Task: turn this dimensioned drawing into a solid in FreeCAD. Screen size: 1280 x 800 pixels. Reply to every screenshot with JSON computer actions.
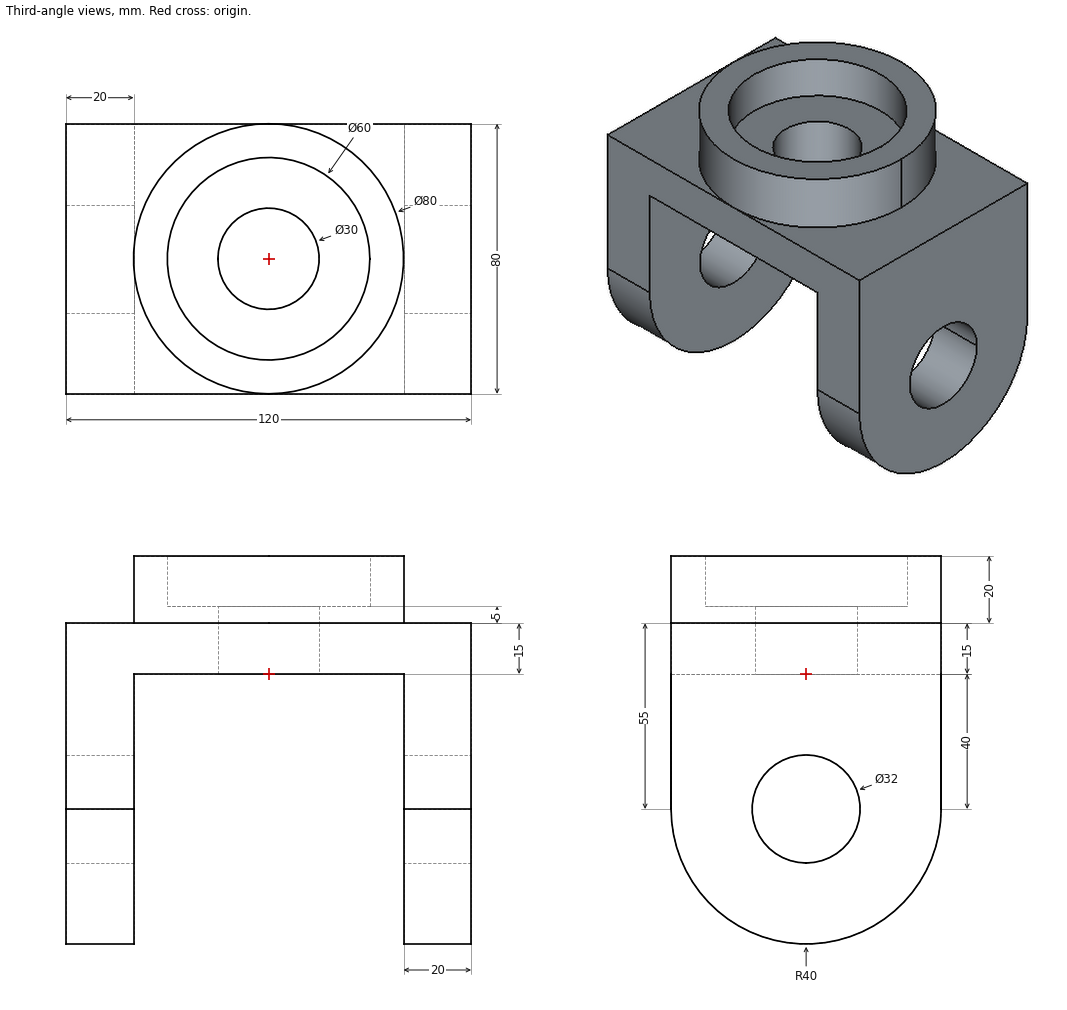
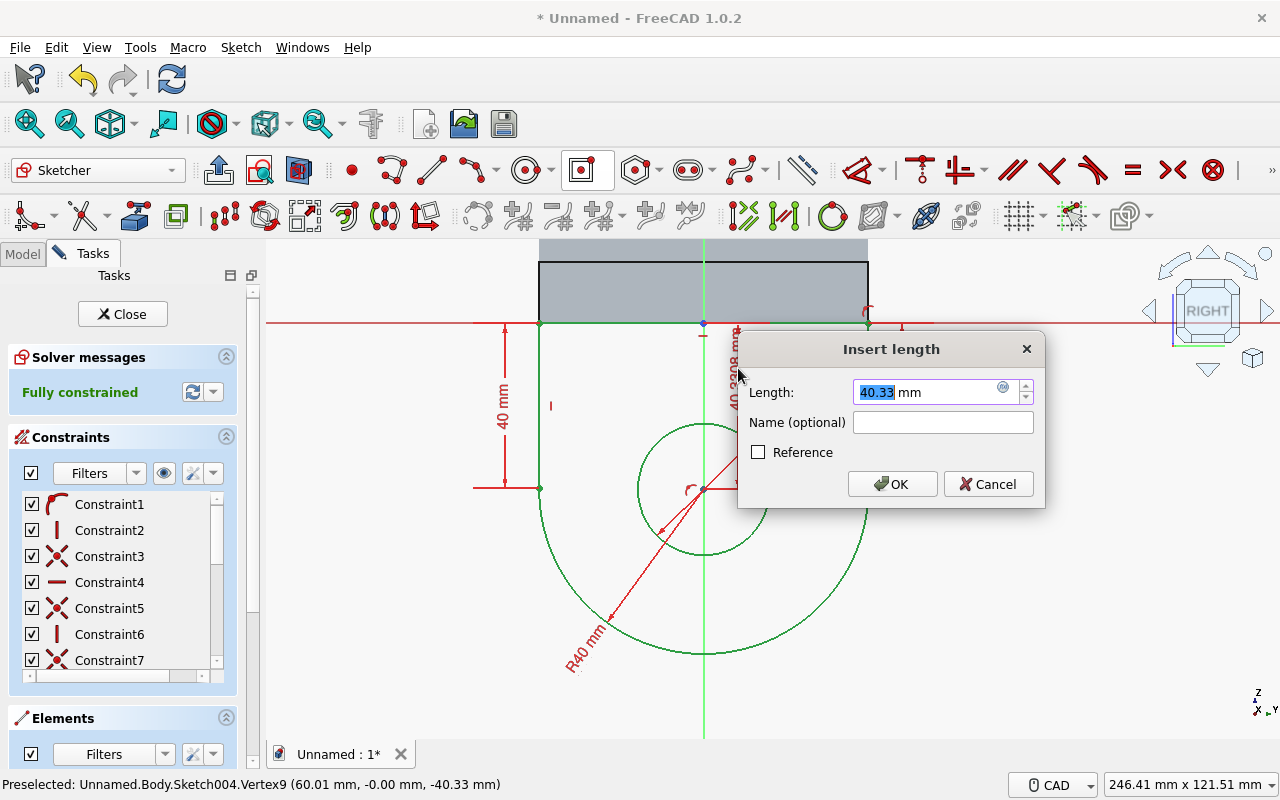
{"action": "type", "text": "40"}
{"action": "key", "text": "Return"}
{"action": "key", "text": "Escape"}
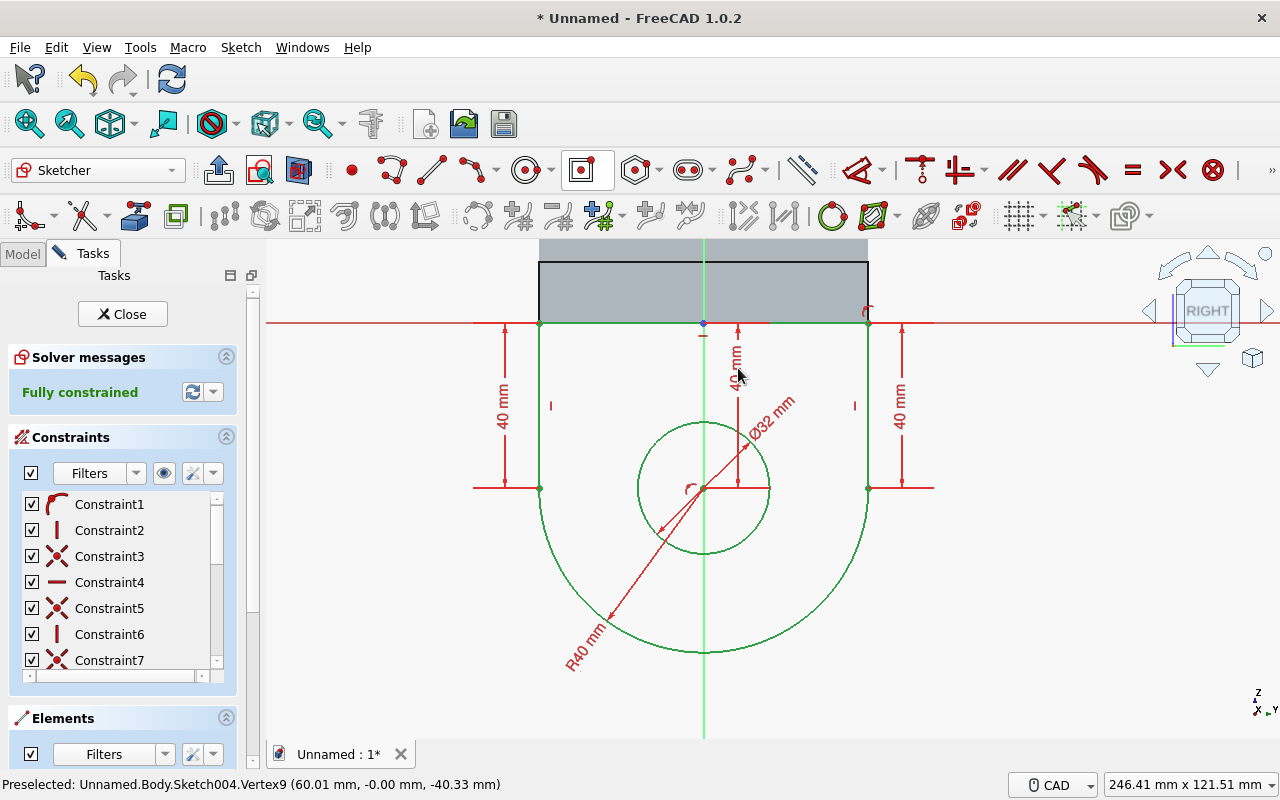
{"action": "left_click", "coordinate": [123, 314]}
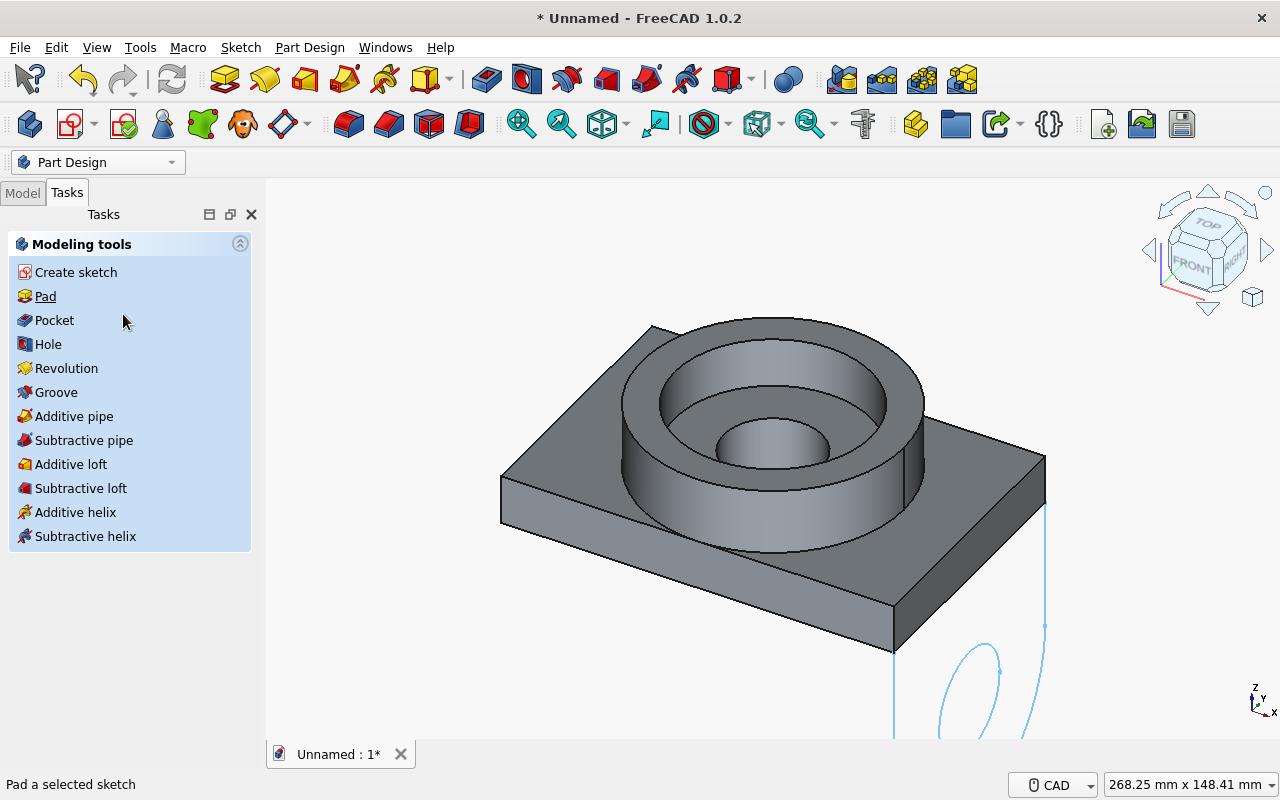
{"action": "left_click", "coordinate": [226, 80]}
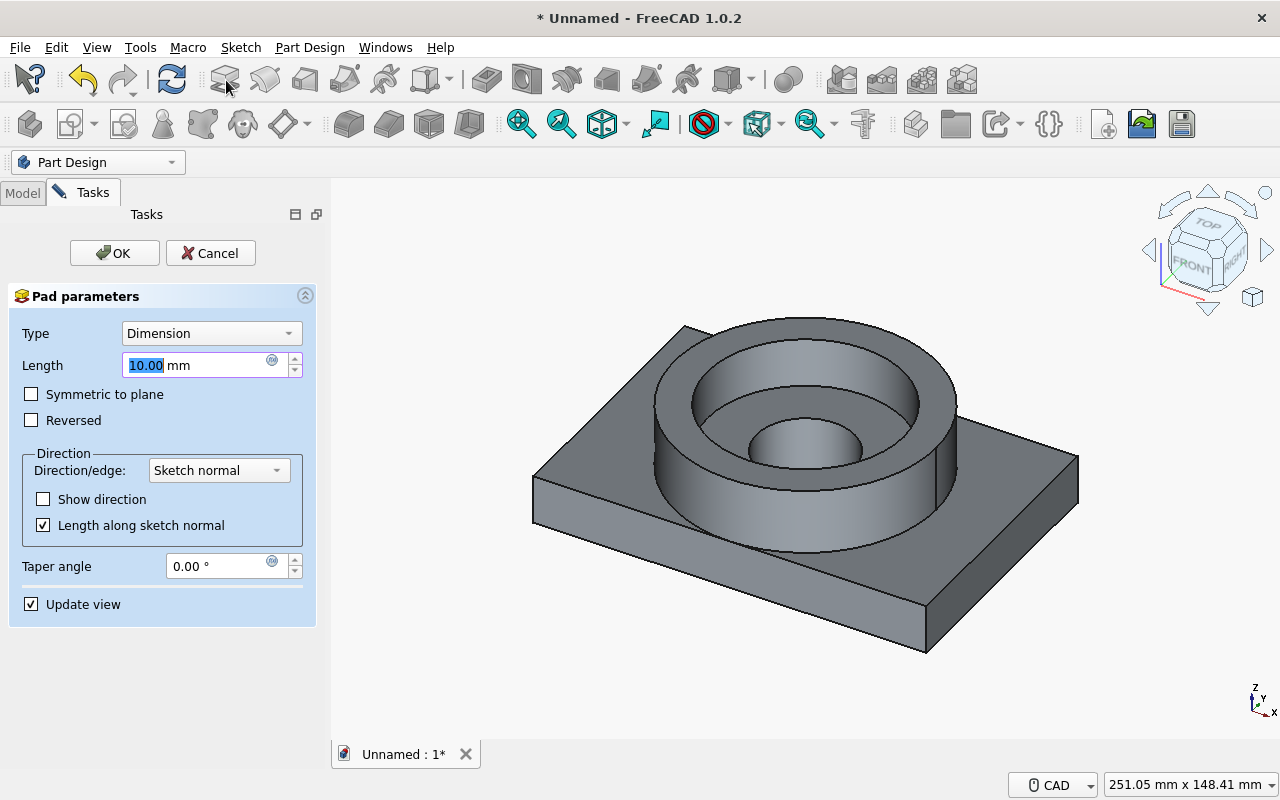
{"action": "type", "text": "20"}
{"action": "key", "text": "Tab"}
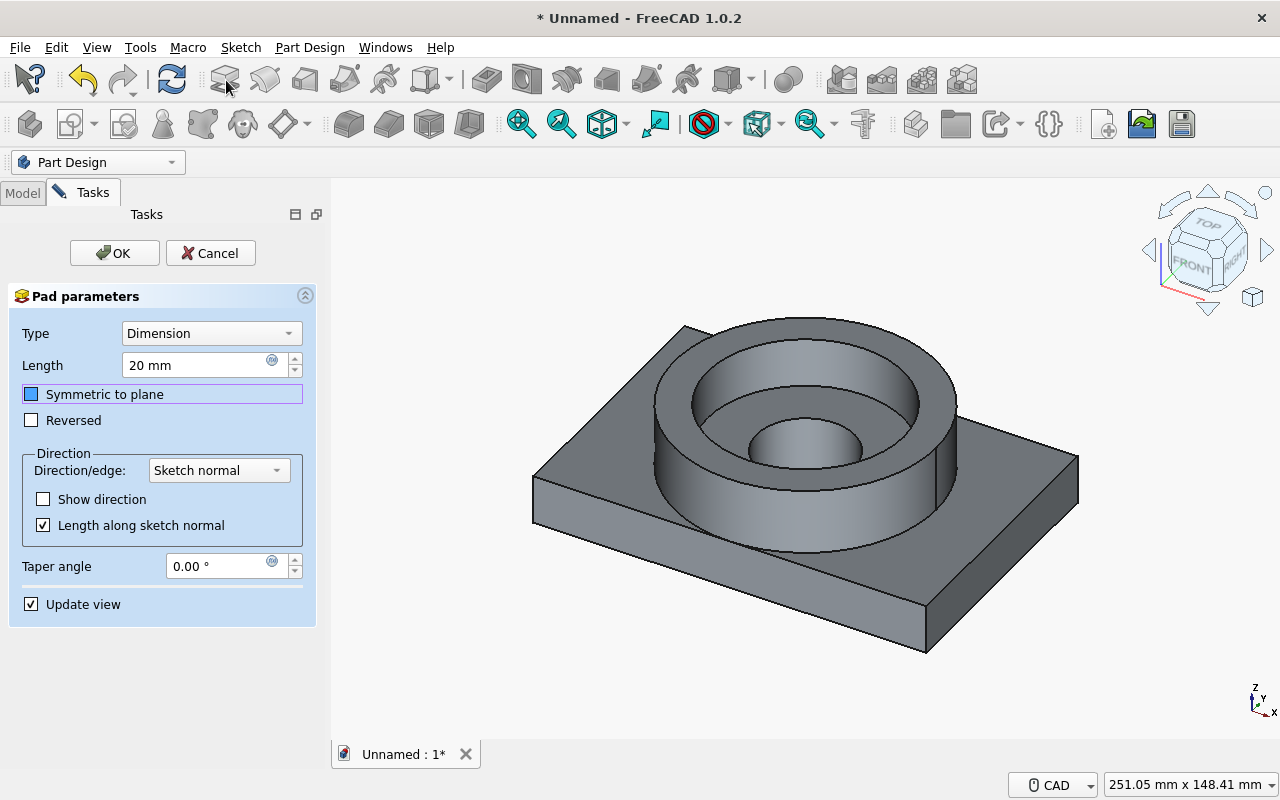
{"action": "left_click", "coordinate": [30, 420]}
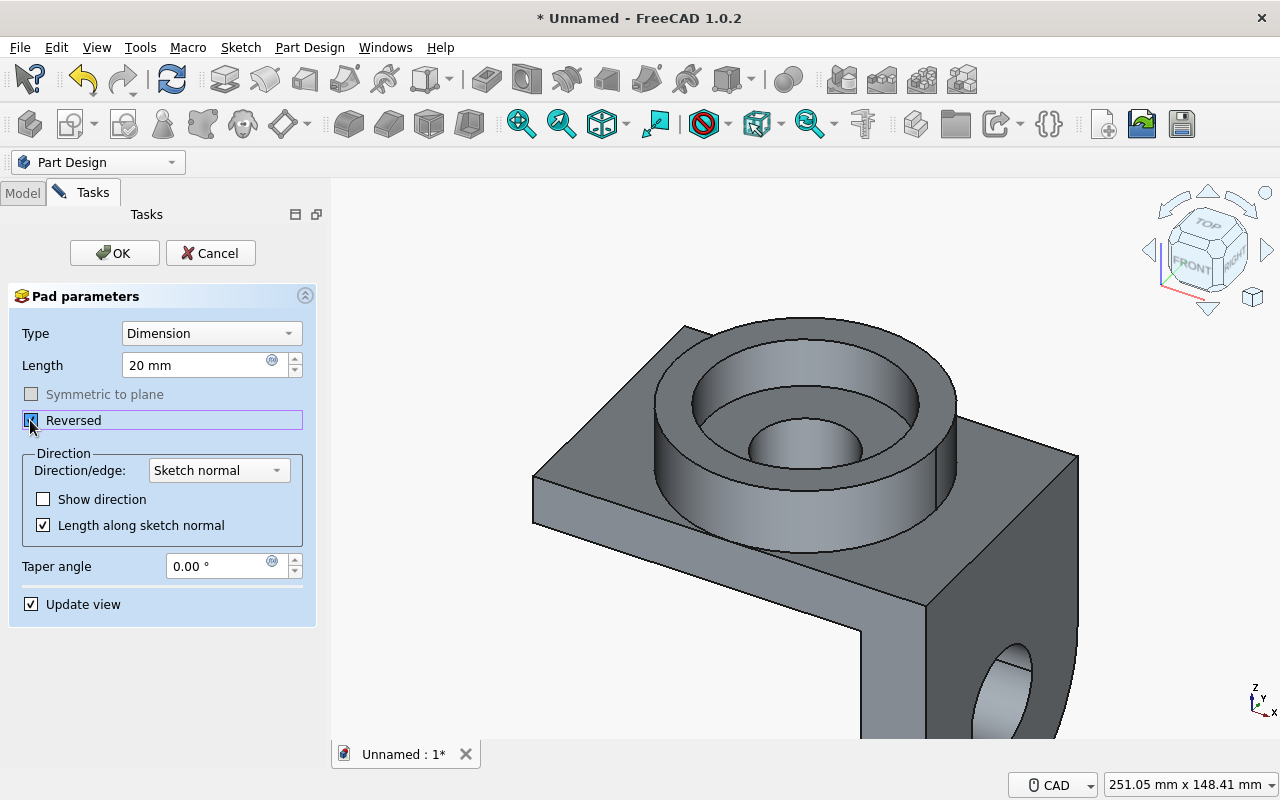
{"action": "left_click", "coordinate": [115, 253]}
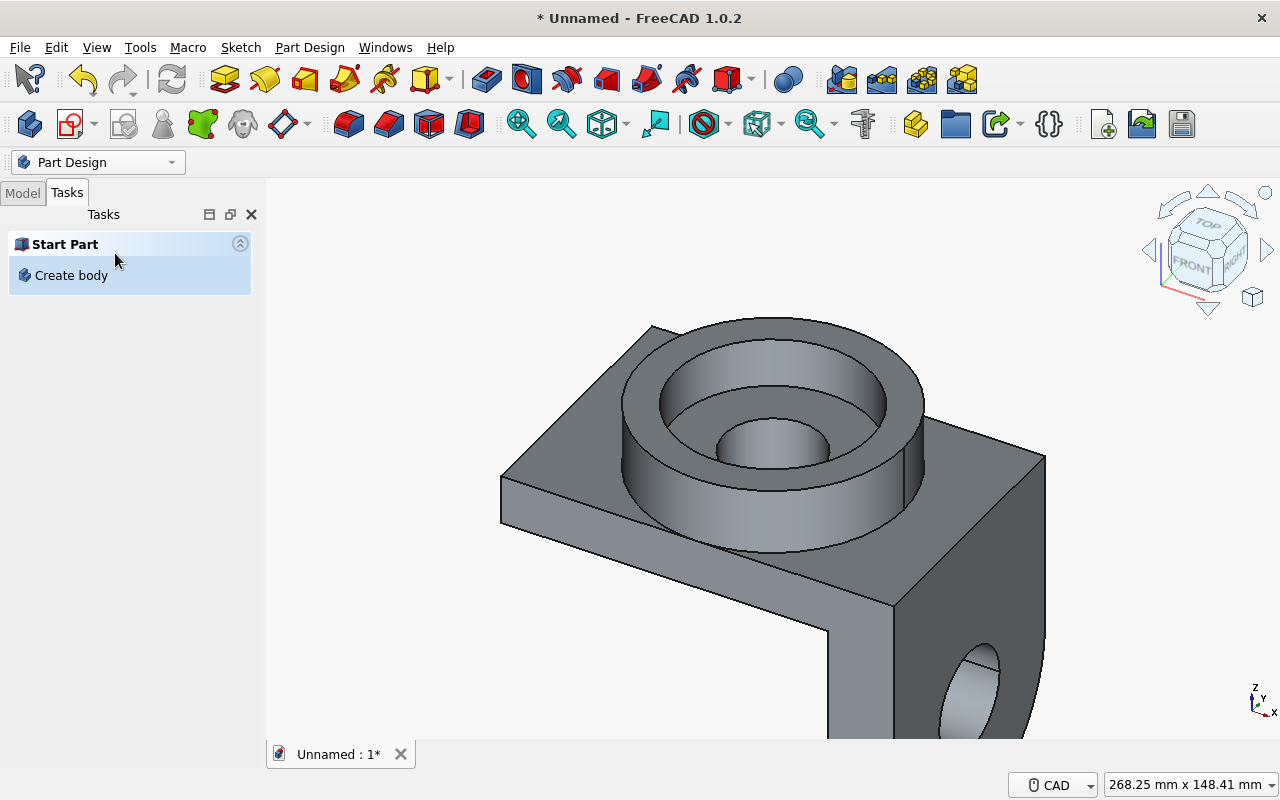
{"action": "left_click", "coordinate": [522, 124]}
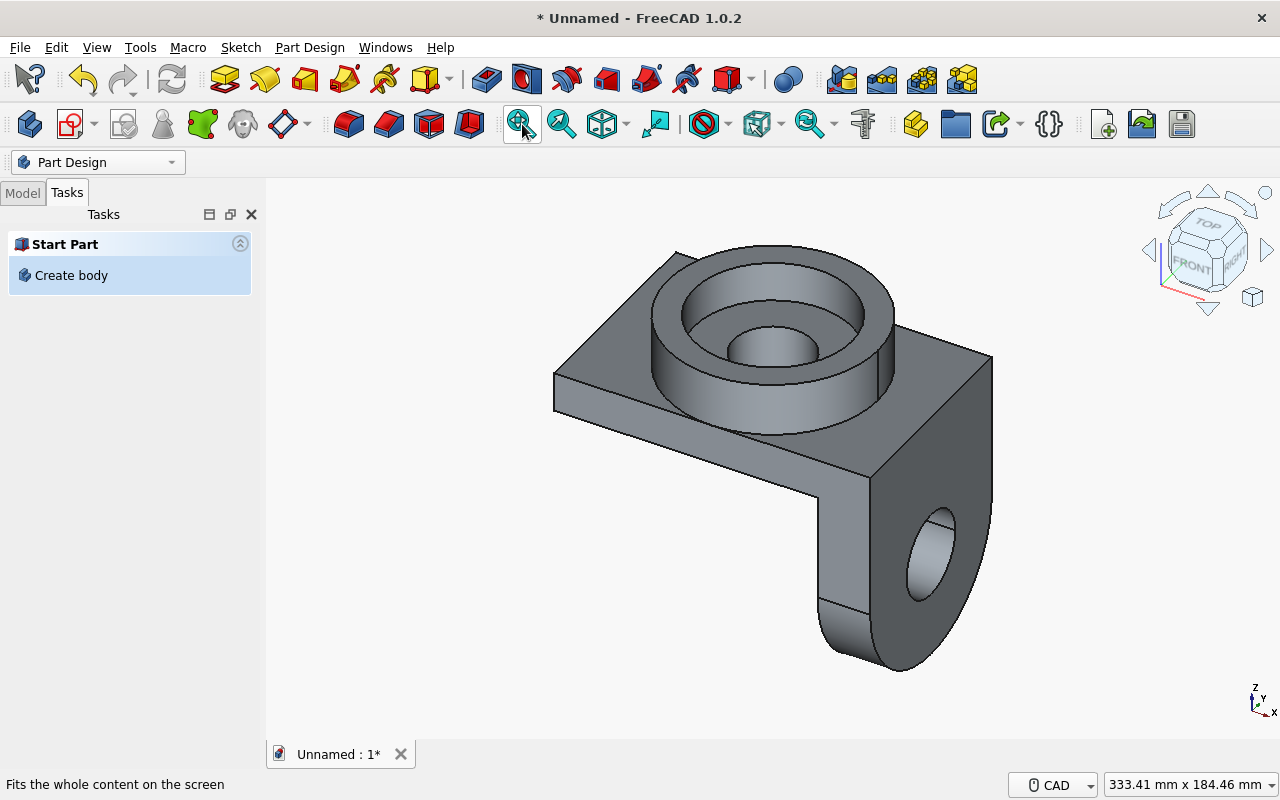
{"action": "left_click", "coordinate": [23, 192]}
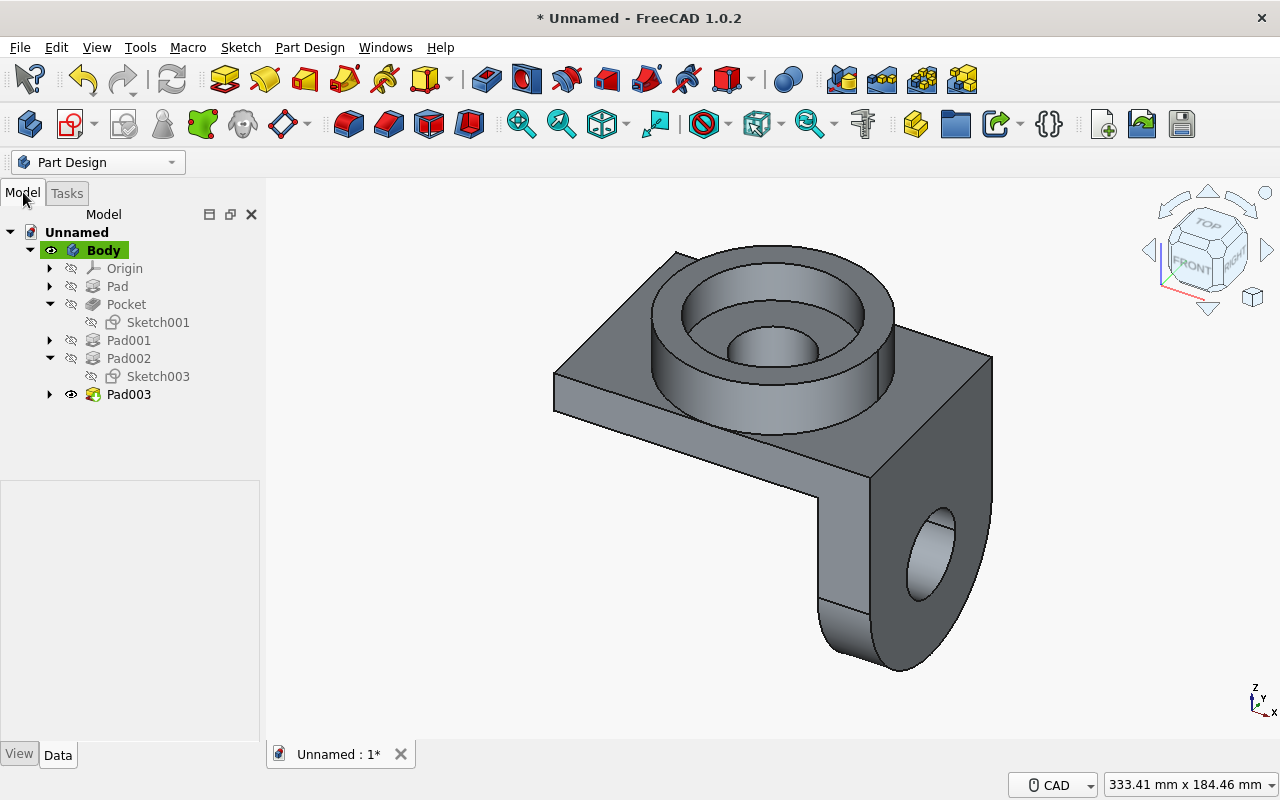
{"action": "left_click", "coordinate": [50, 268]}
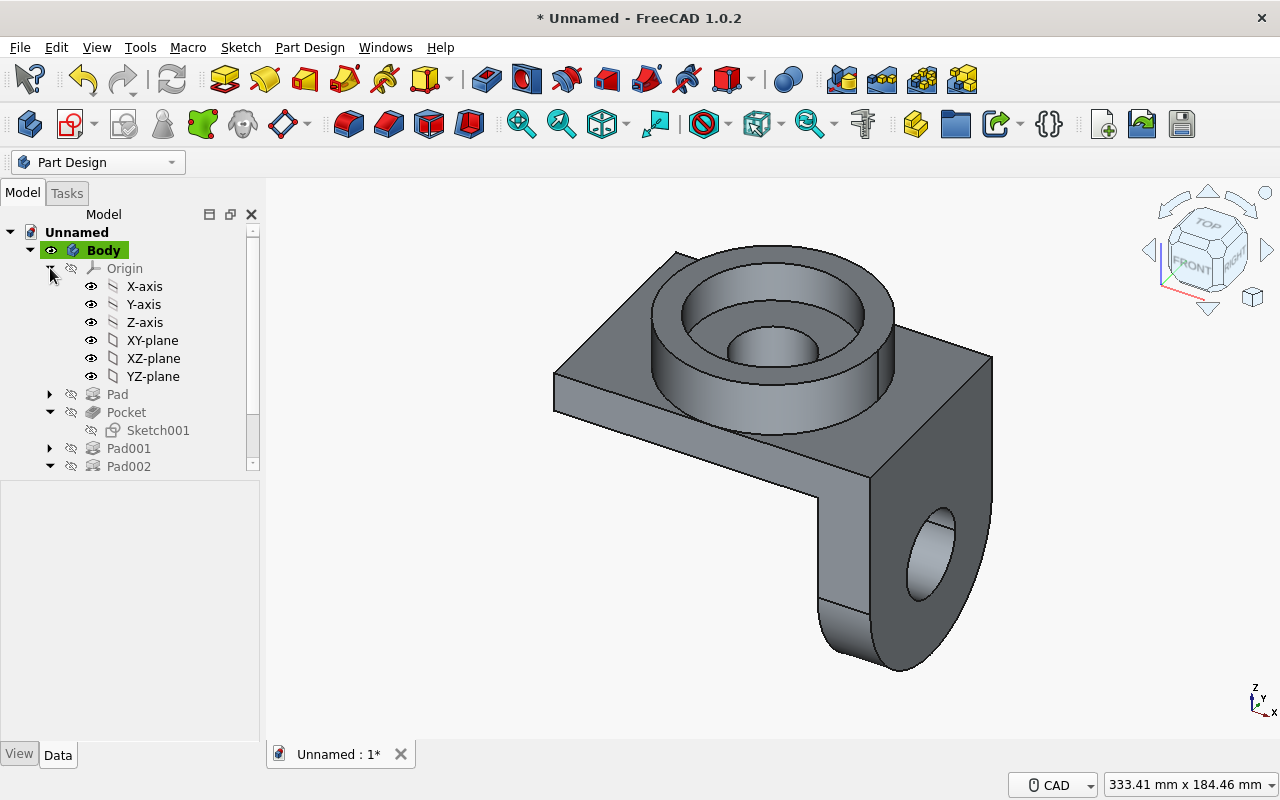
{"action": "left_click", "coordinate": [136, 376]}